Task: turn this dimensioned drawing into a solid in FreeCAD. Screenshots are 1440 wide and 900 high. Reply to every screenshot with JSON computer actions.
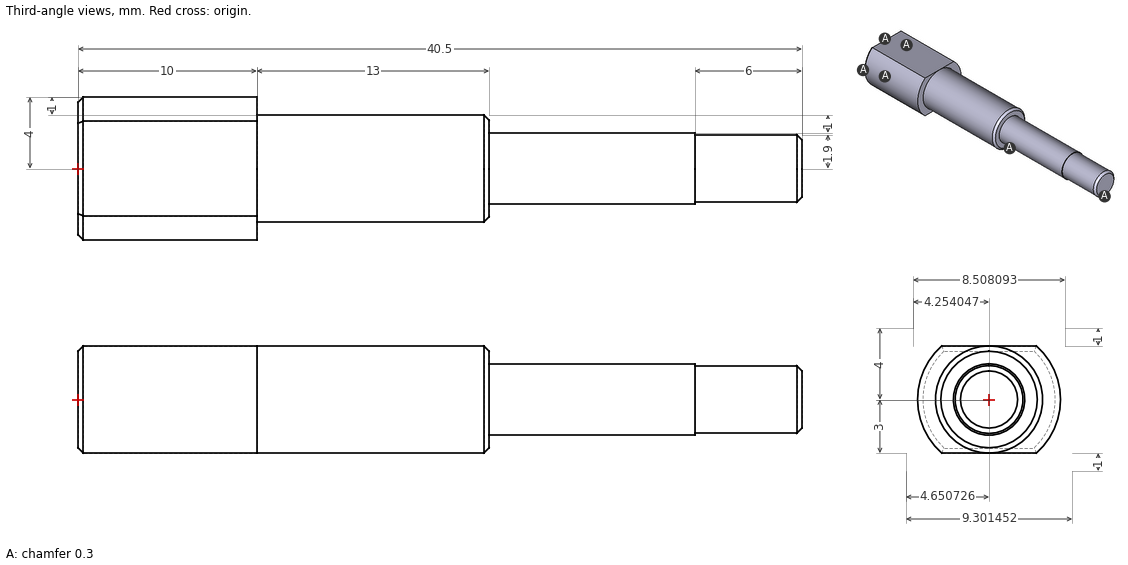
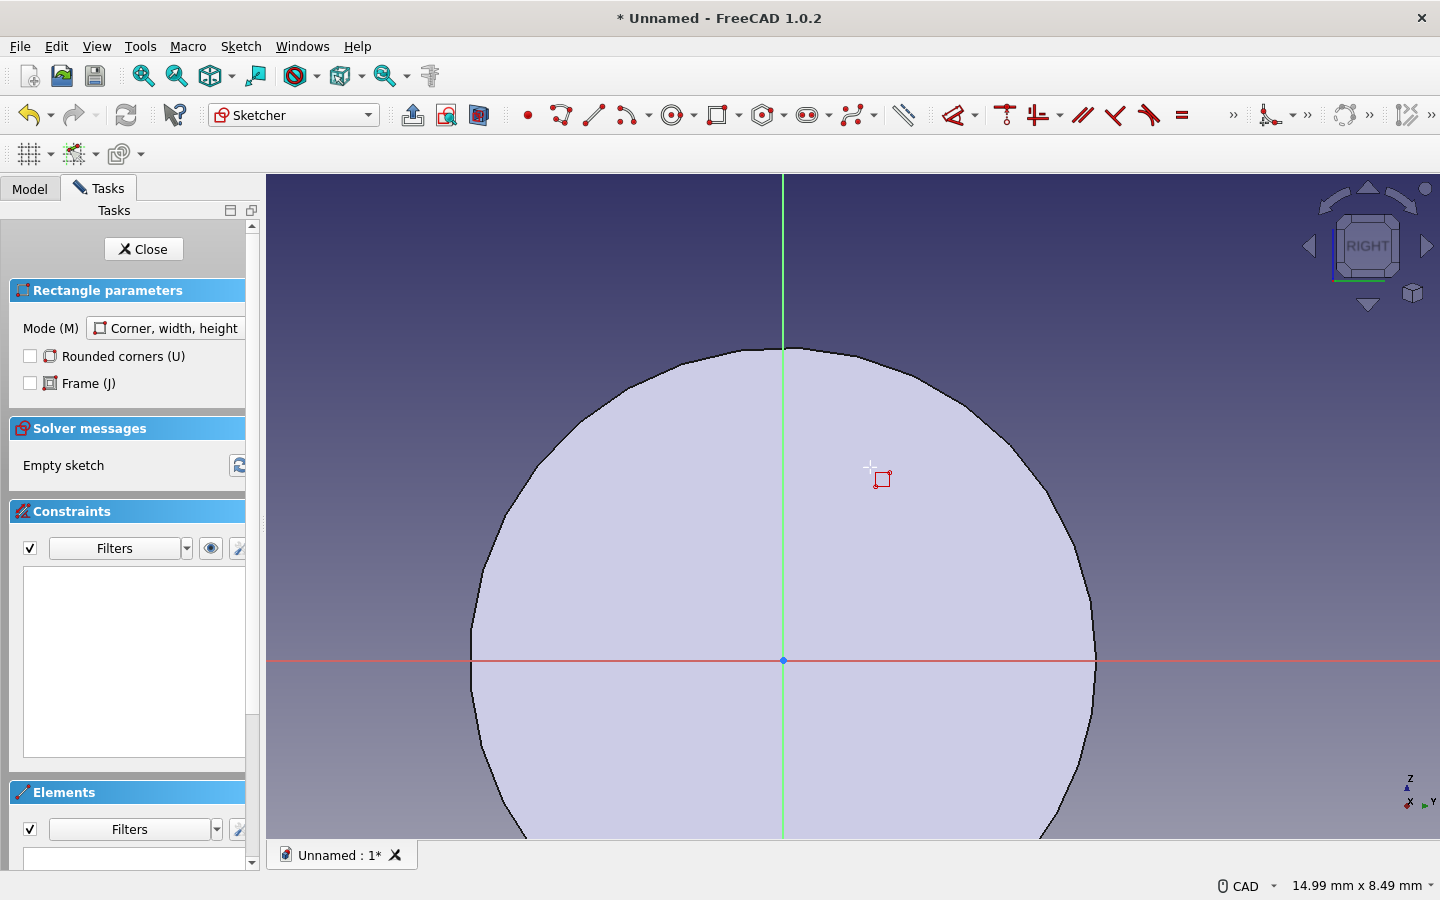
{"action": "left_click", "coordinate": [450, 348]}
{"action": "mouse_move", "coordinate": [1116, 426]}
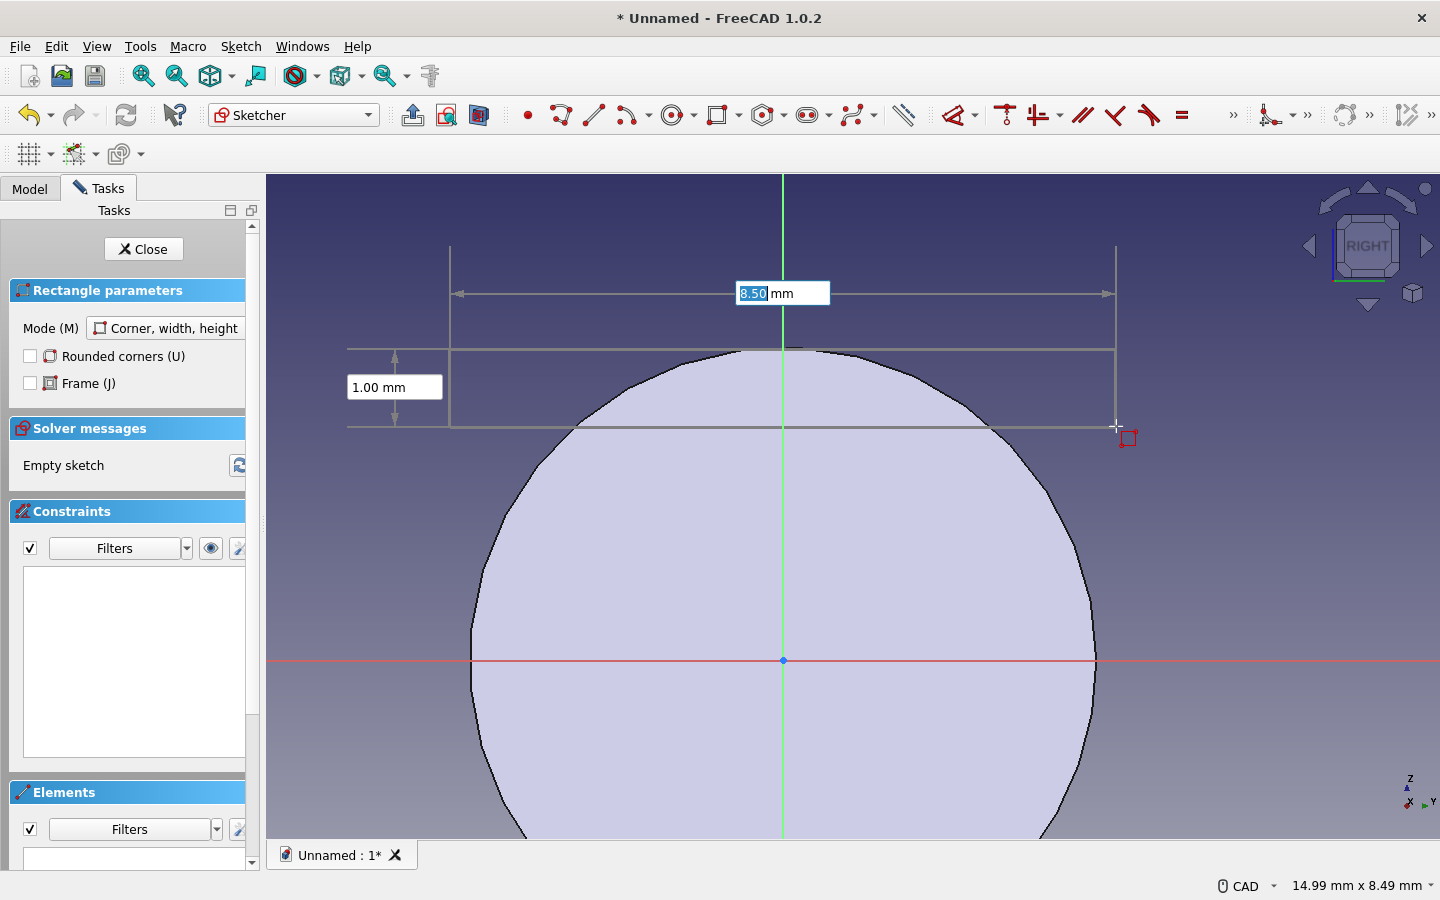
{"action": "type", "text": "8.508093"}
{"action": "key", "text": "Tab"}
{"action": "type", "text": "1"}
{"action": "key", "text": "Return"}
{"action": "key", "text": "Escape"}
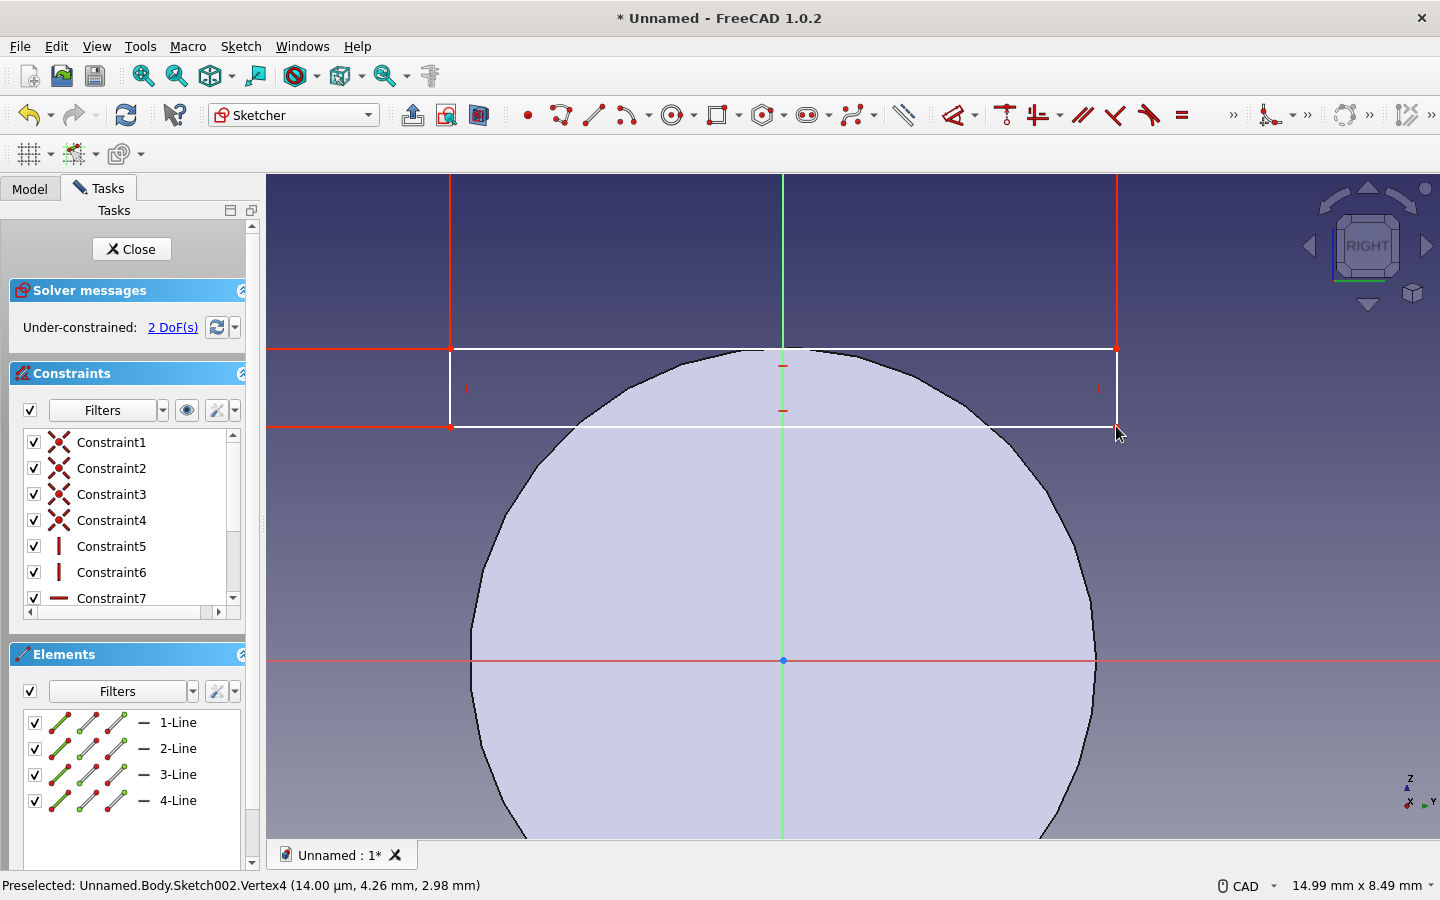
{"action": "key", "text": "d"}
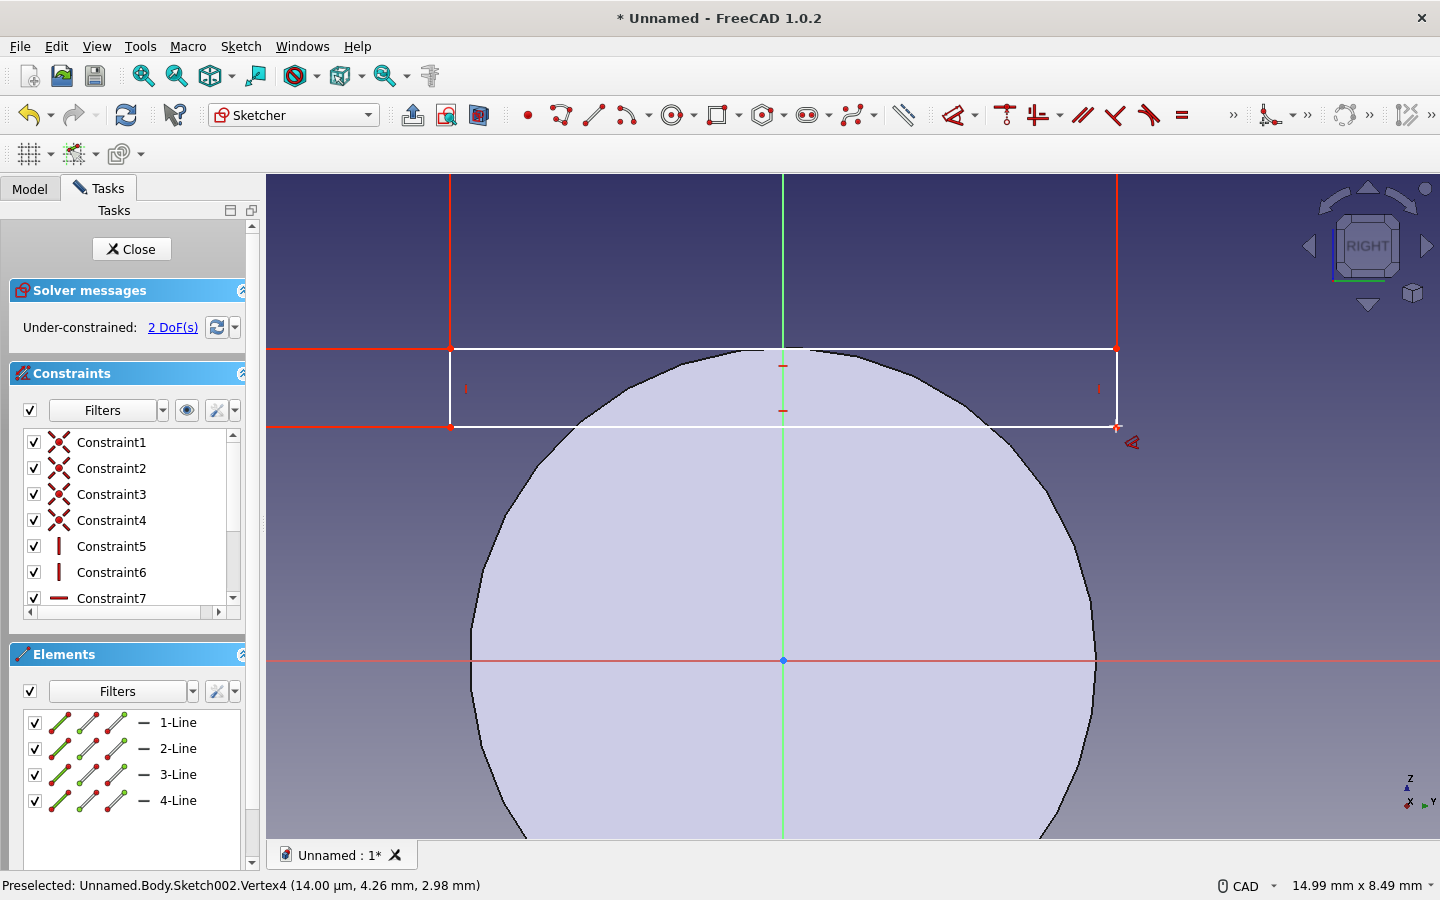
{"action": "left_click", "coordinate": [450, 349]}
{"action": "left_click", "coordinate": [416, 505]}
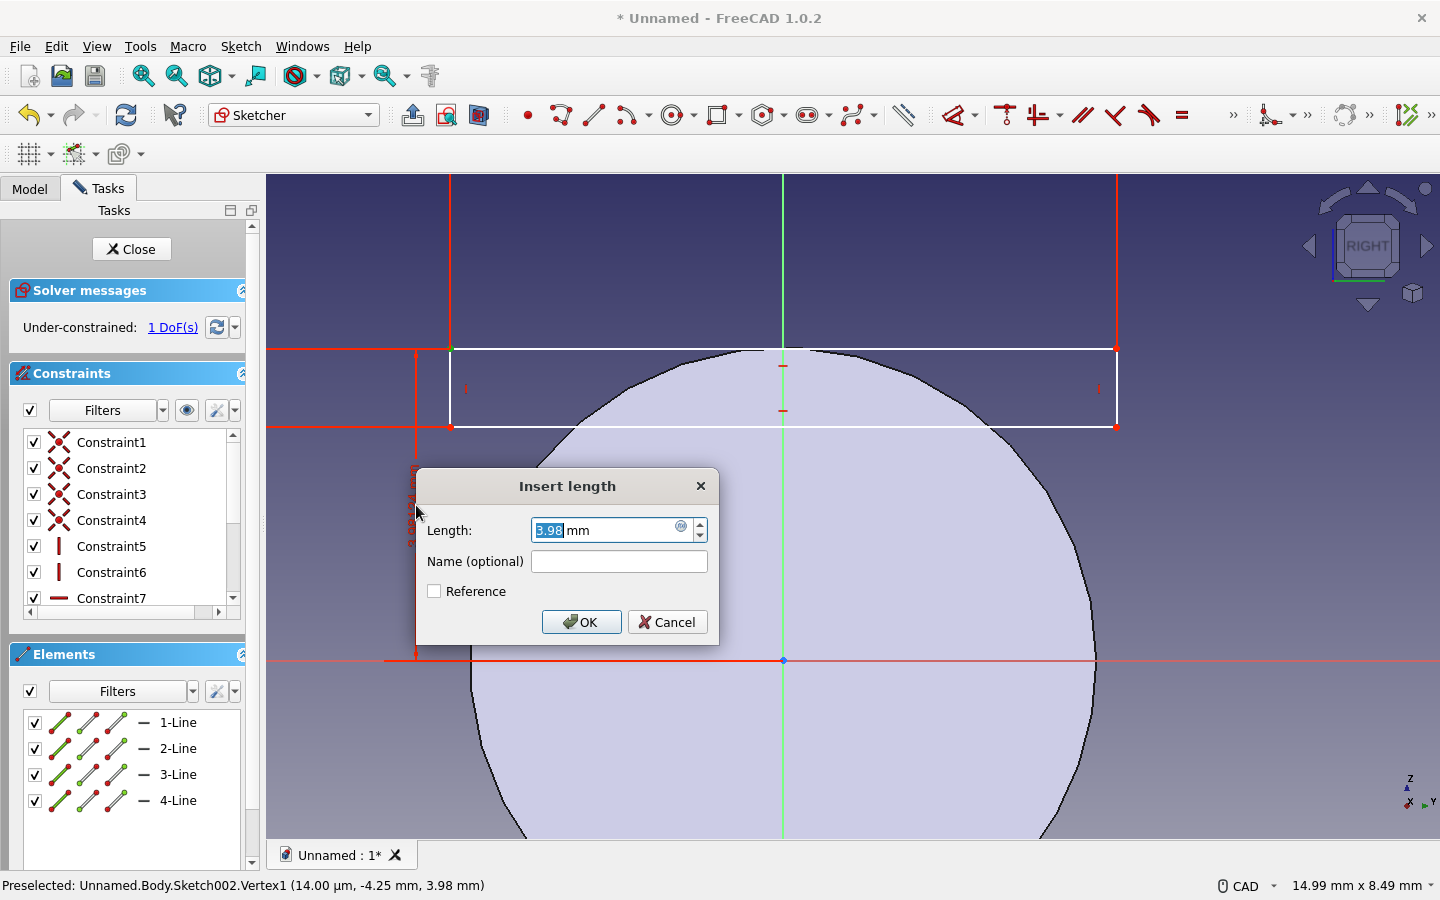
{"action": "type", "text": "4"}
{"action": "key", "text": "Return"}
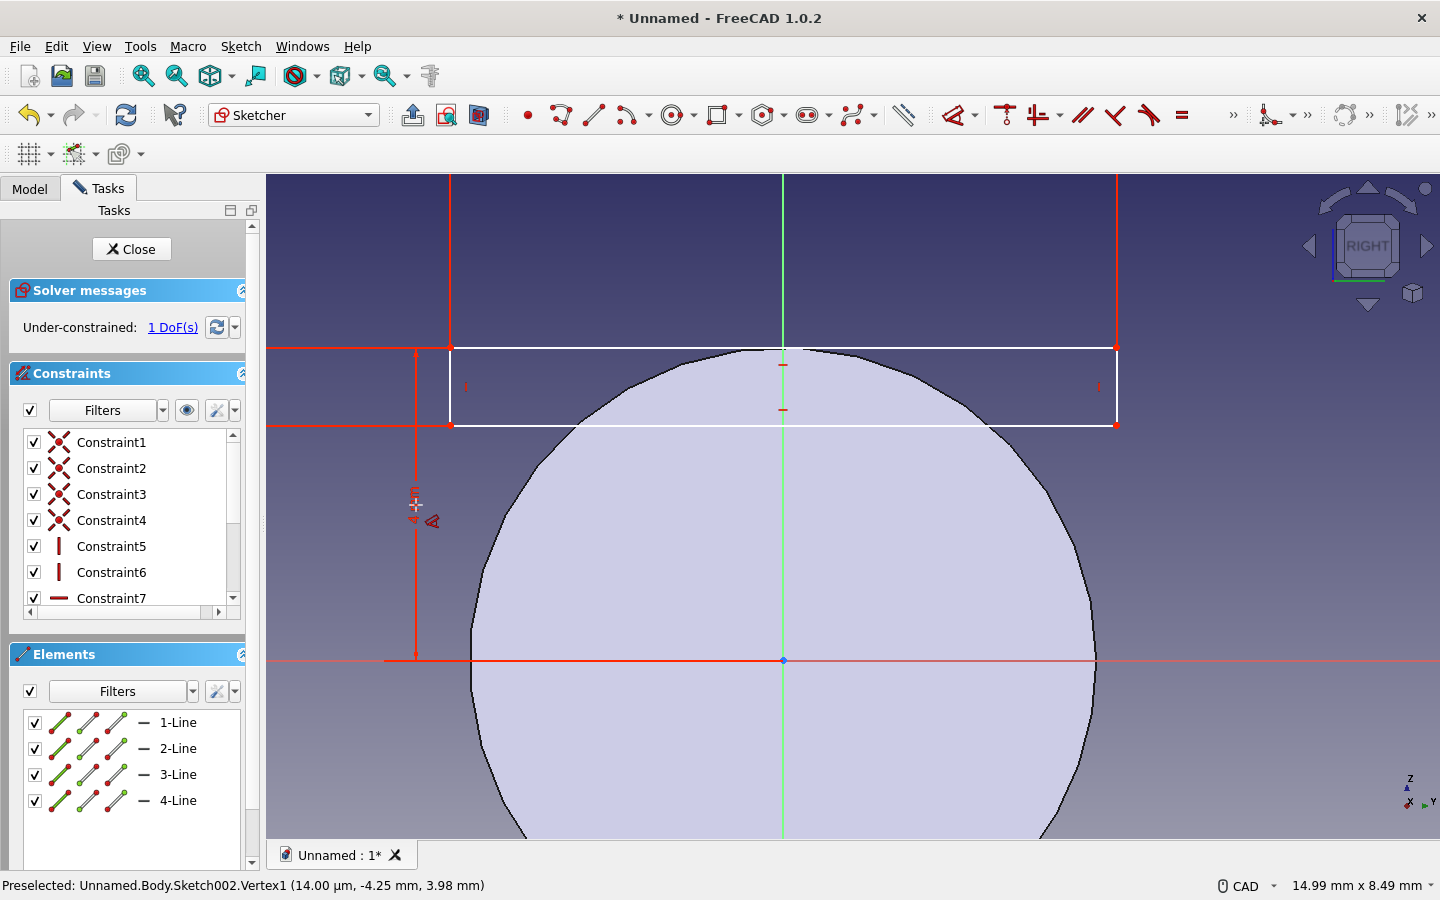
{"action": "left_click", "coordinate": [450, 348]}
{"action": "left_click", "coordinate": [617, 695]}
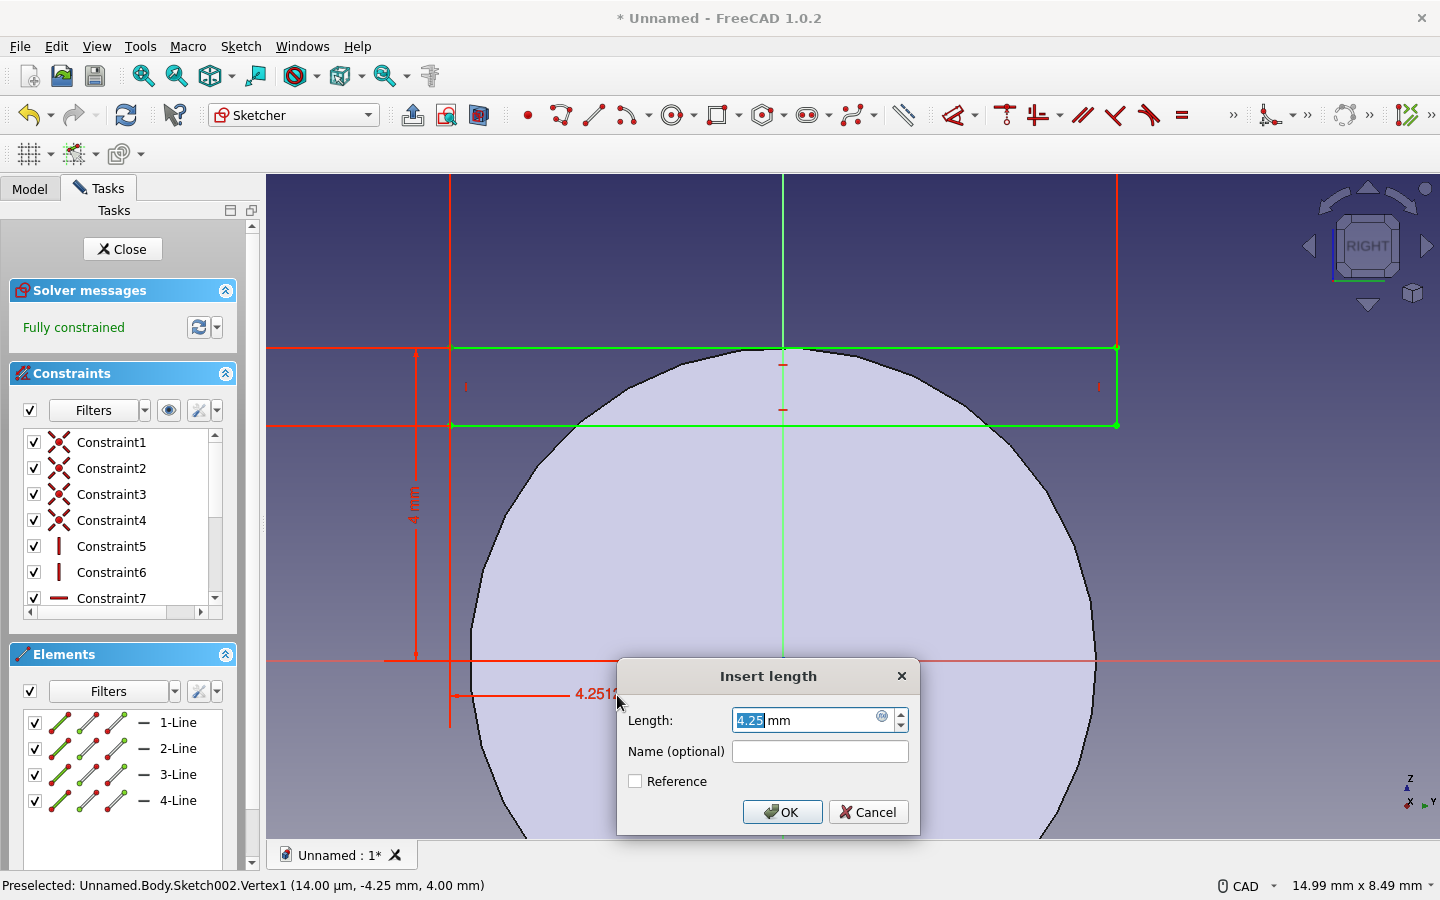
{"action": "type", "text": "4.254047"}
{"action": "key", "text": "Return"}
{"action": "key", "text": "Escape"}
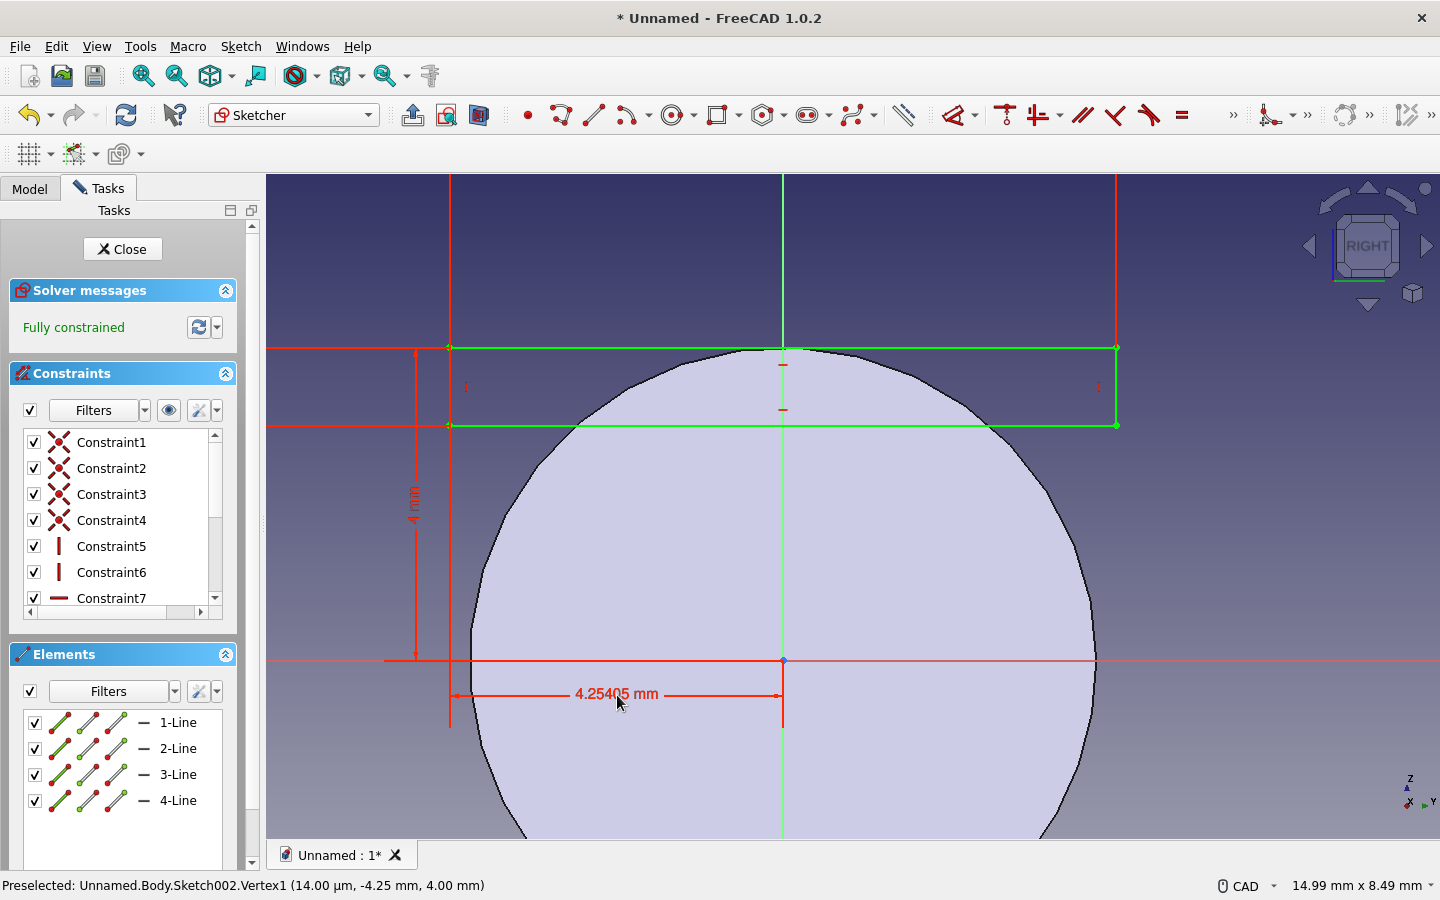
{"action": "left_click", "coordinate": [123, 249]}